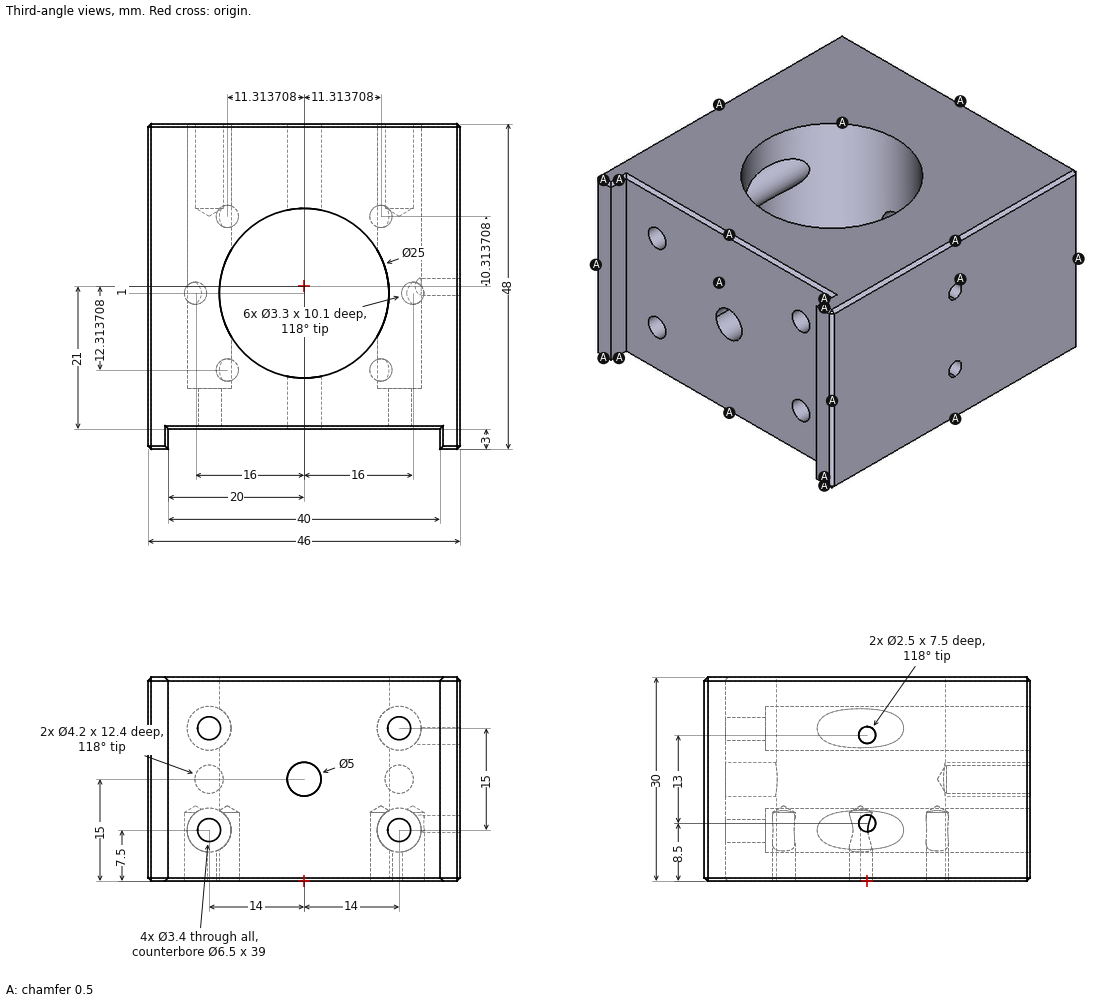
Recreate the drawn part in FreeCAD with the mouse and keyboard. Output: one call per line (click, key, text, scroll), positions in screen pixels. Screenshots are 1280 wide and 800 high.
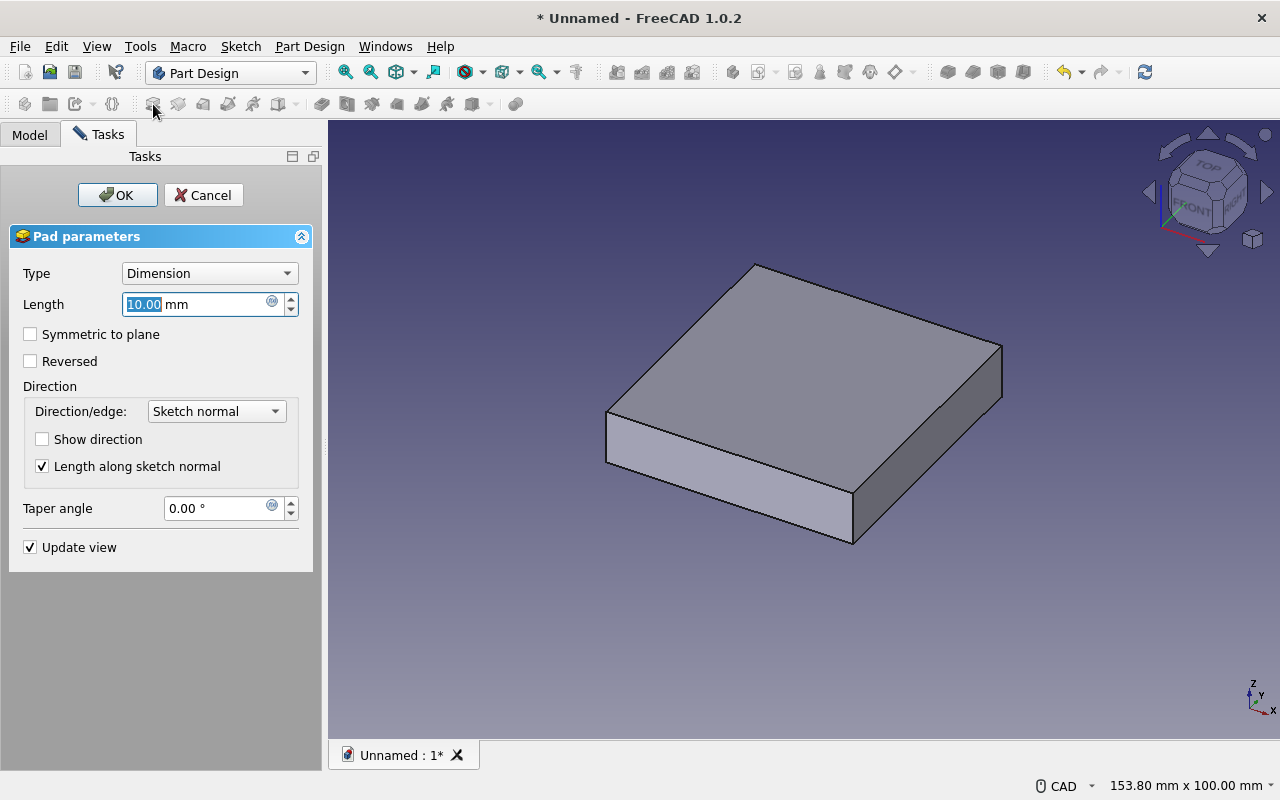
text(30)
key(Tab)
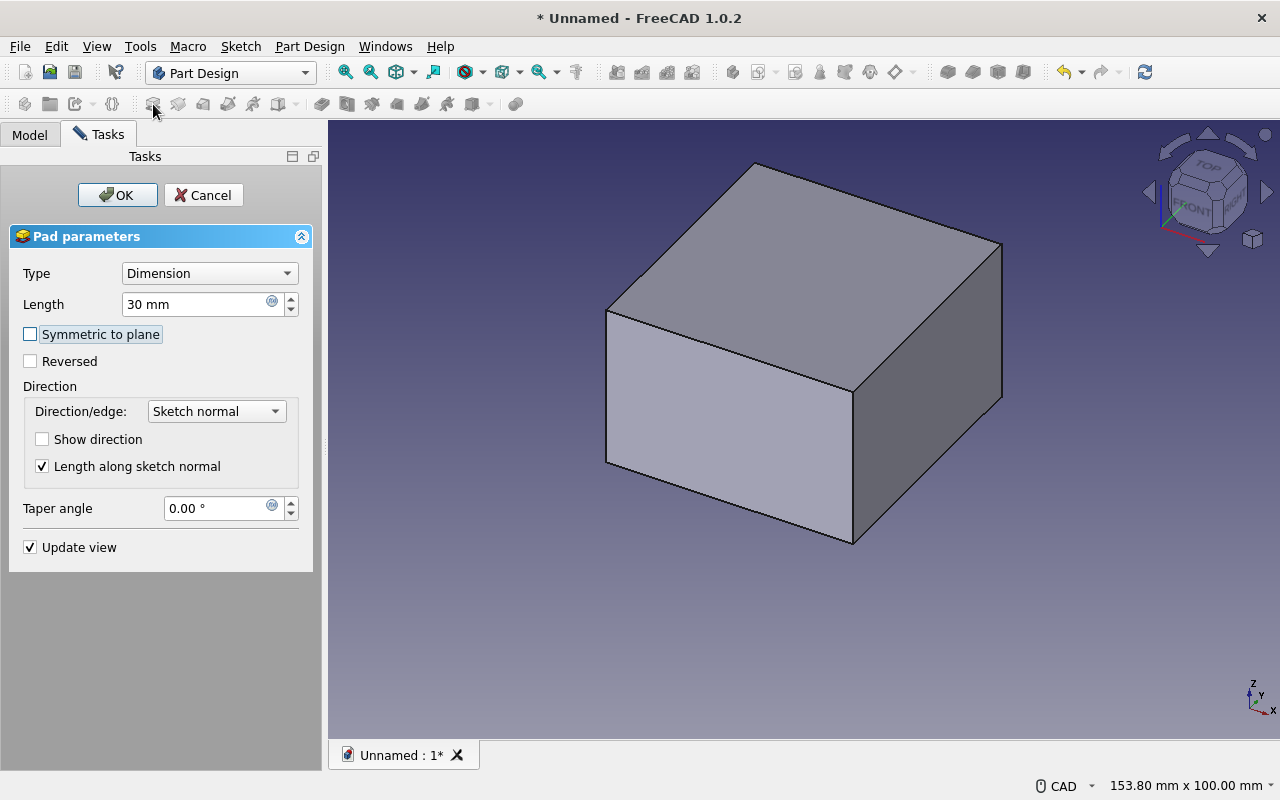
click(118, 195)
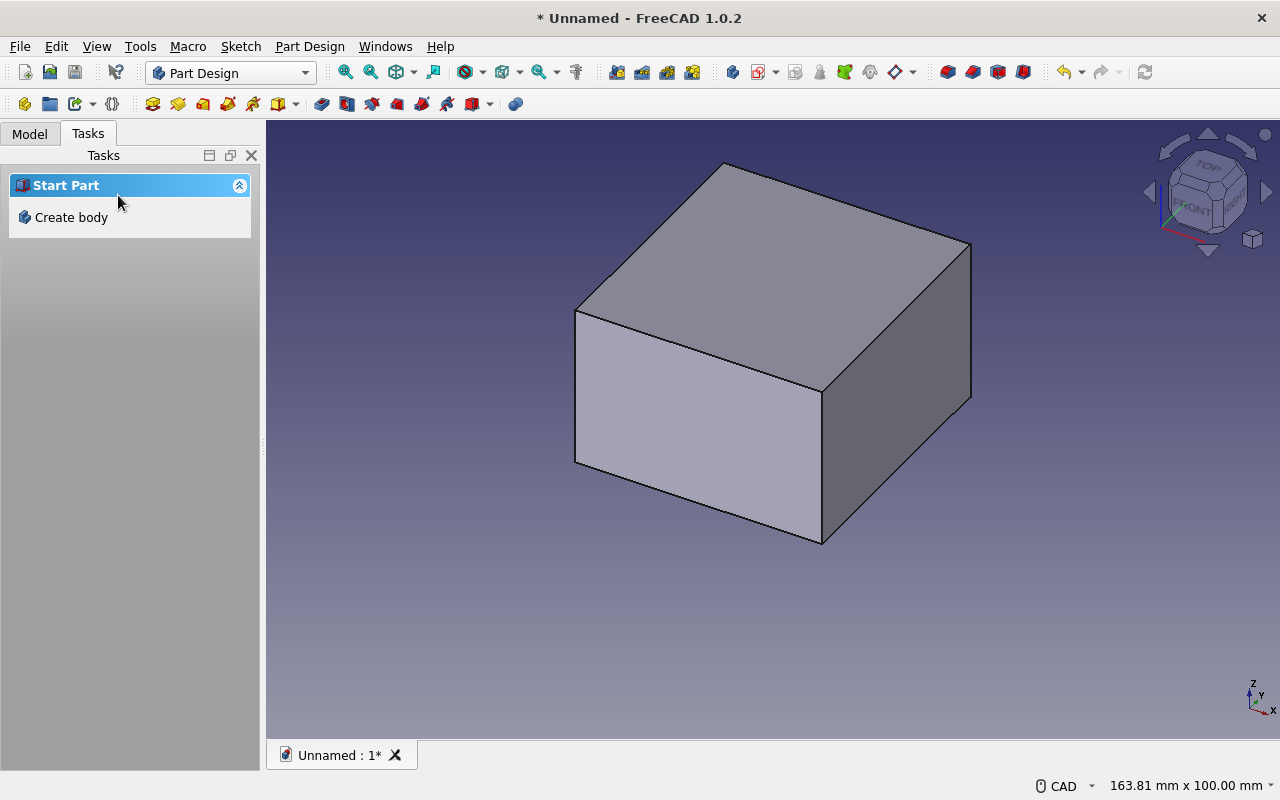
click(773, 276)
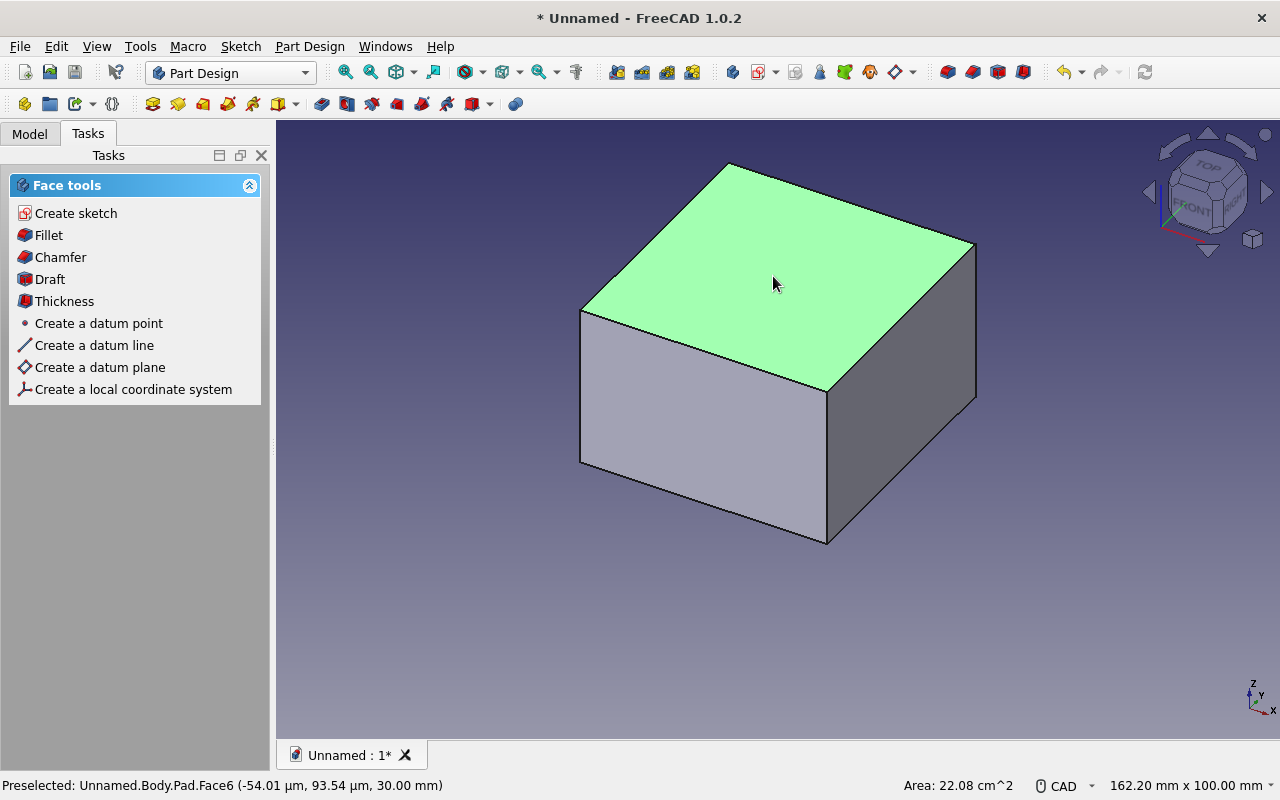
click(758, 72)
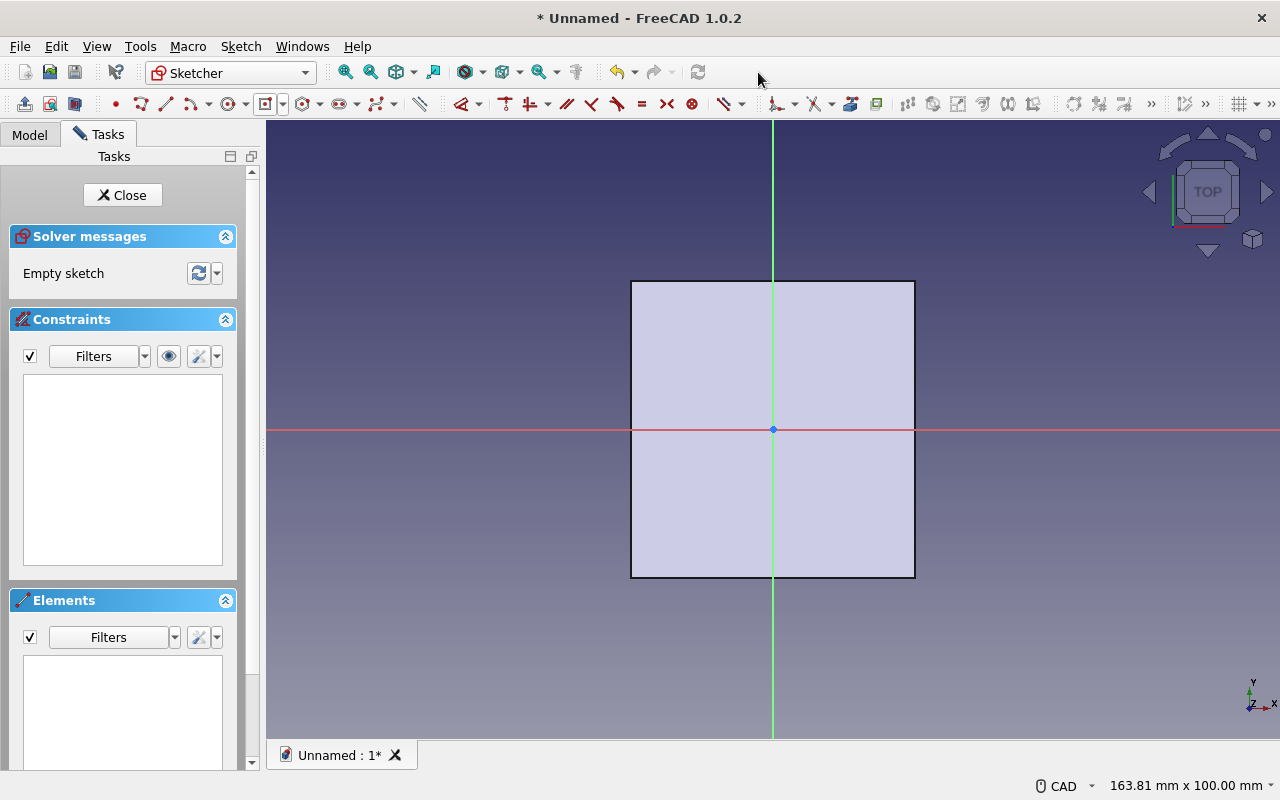
scroll(829, 564, up, 4)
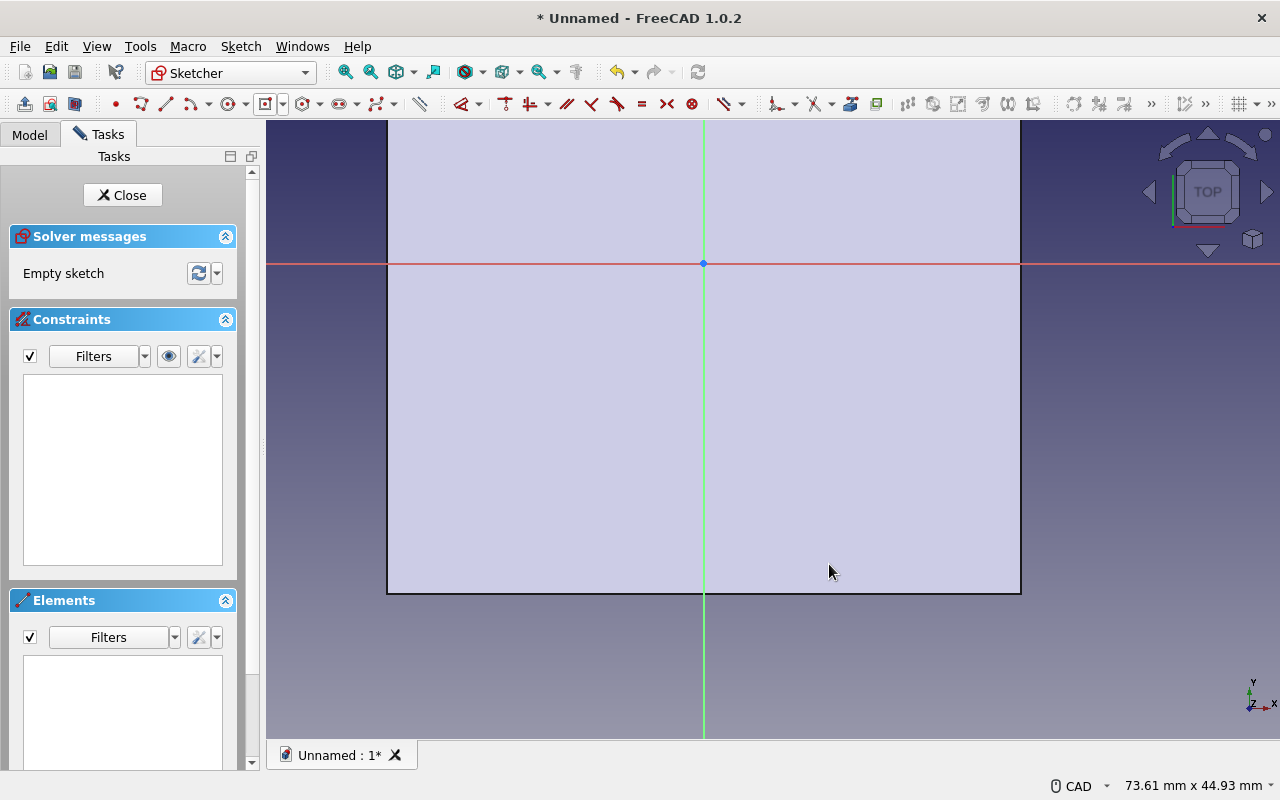
key(g)
key(r)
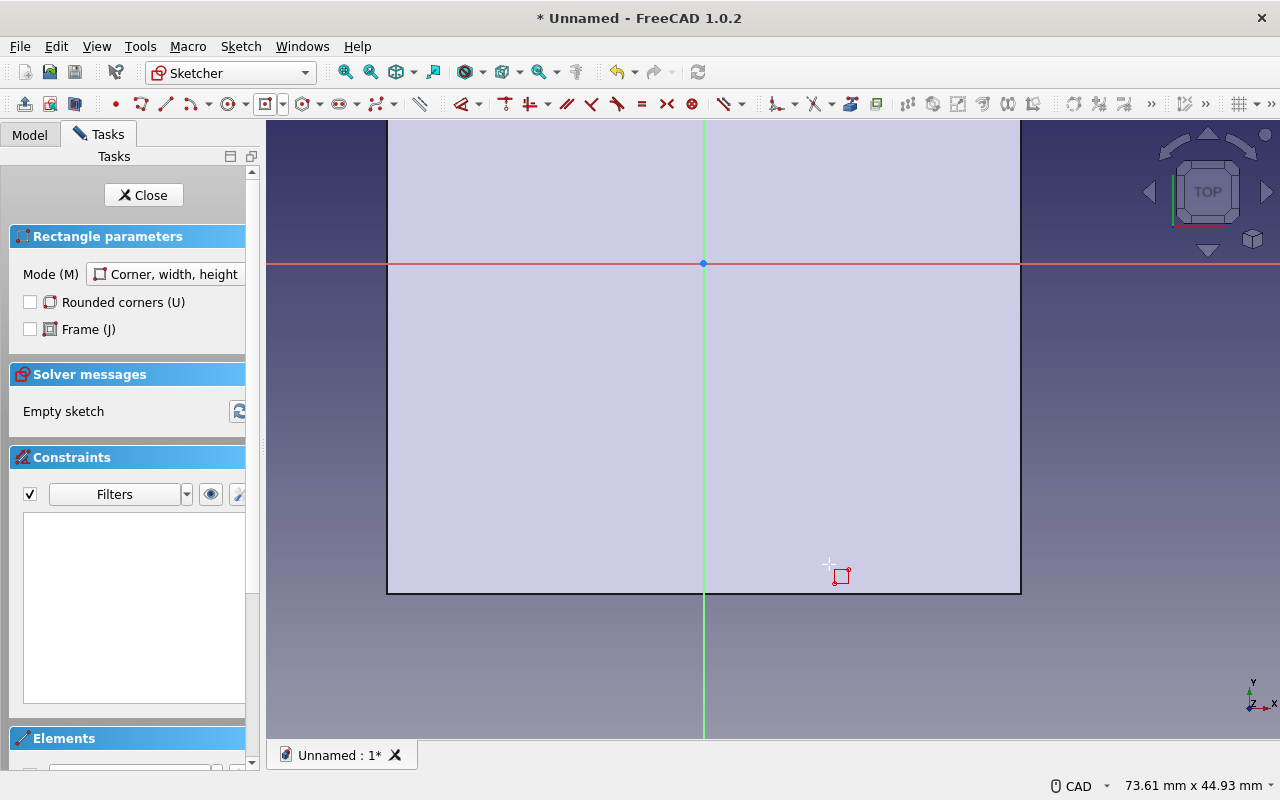
click(428, 553)
move(979, 594)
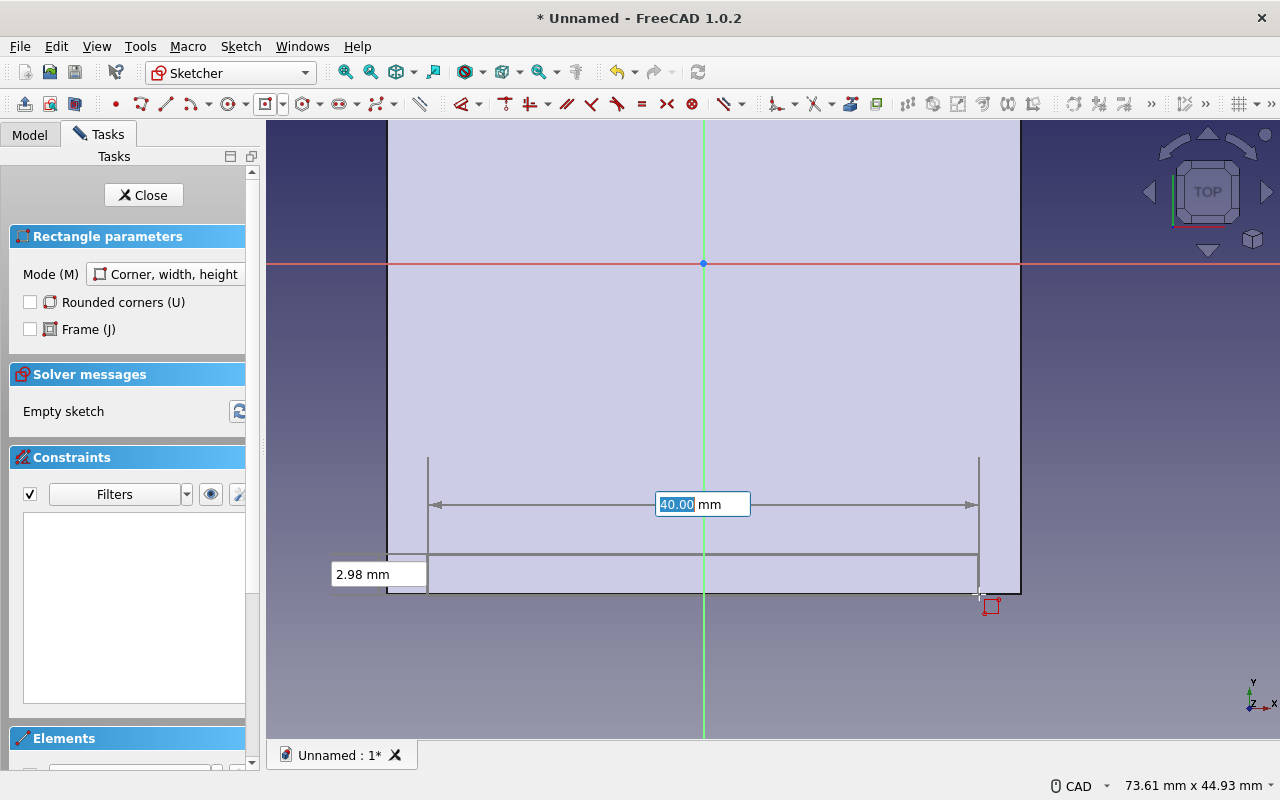
text(40)
key(Tab)
text(3)
key(Return)
key(Escape)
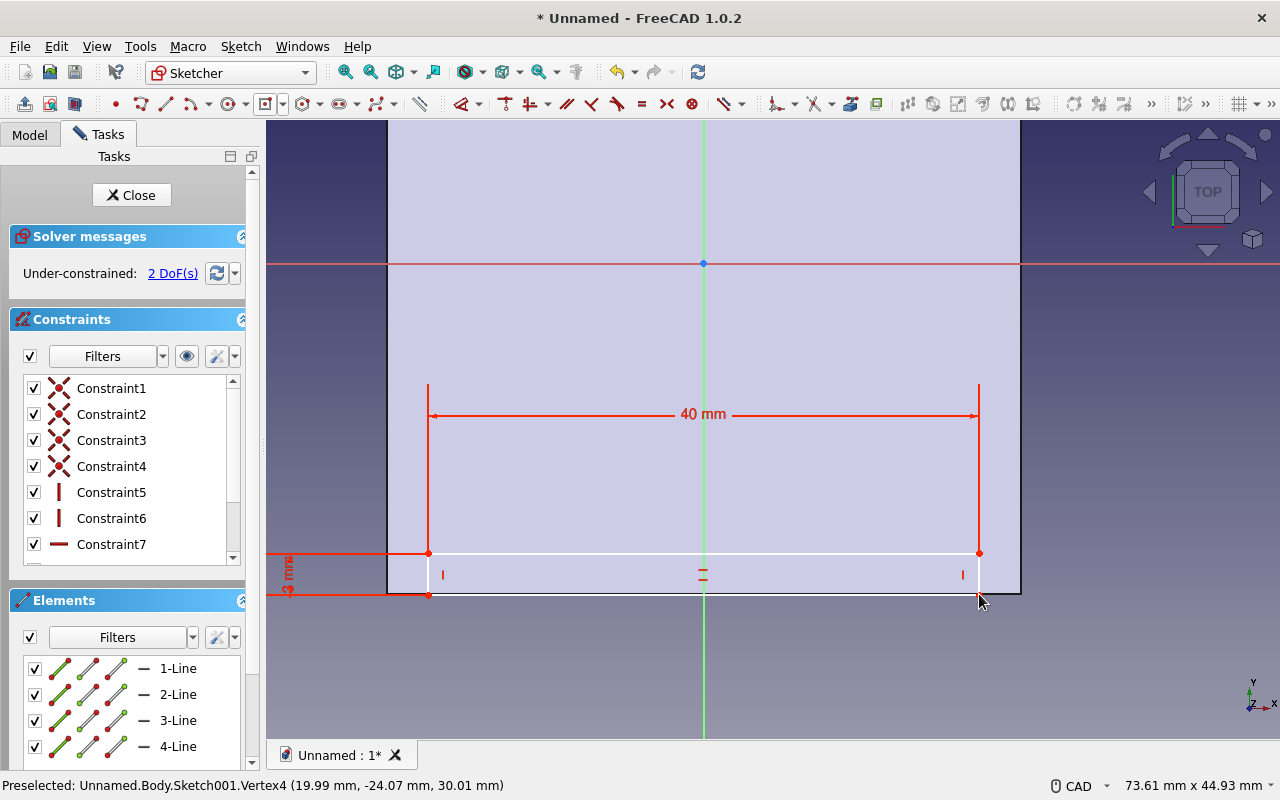
click(460, 104)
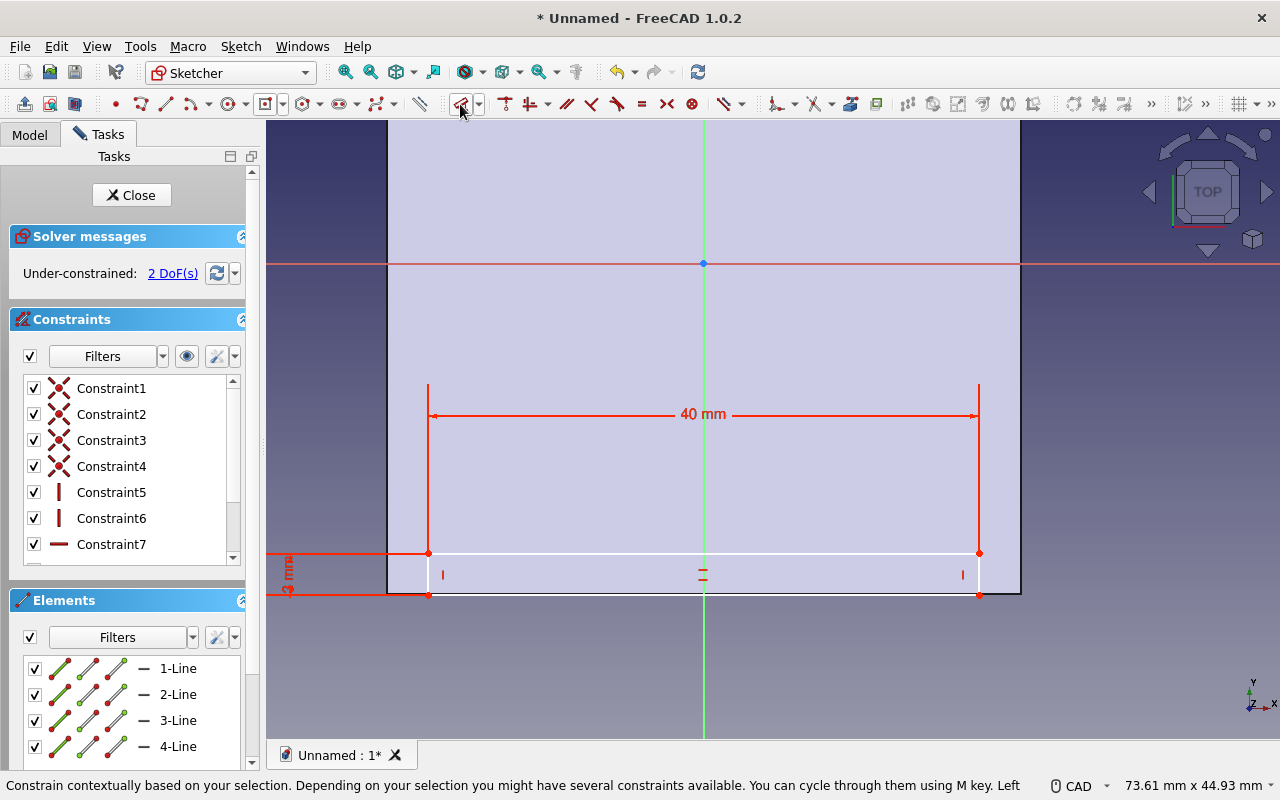
click(428, 554)
click(566, 230)